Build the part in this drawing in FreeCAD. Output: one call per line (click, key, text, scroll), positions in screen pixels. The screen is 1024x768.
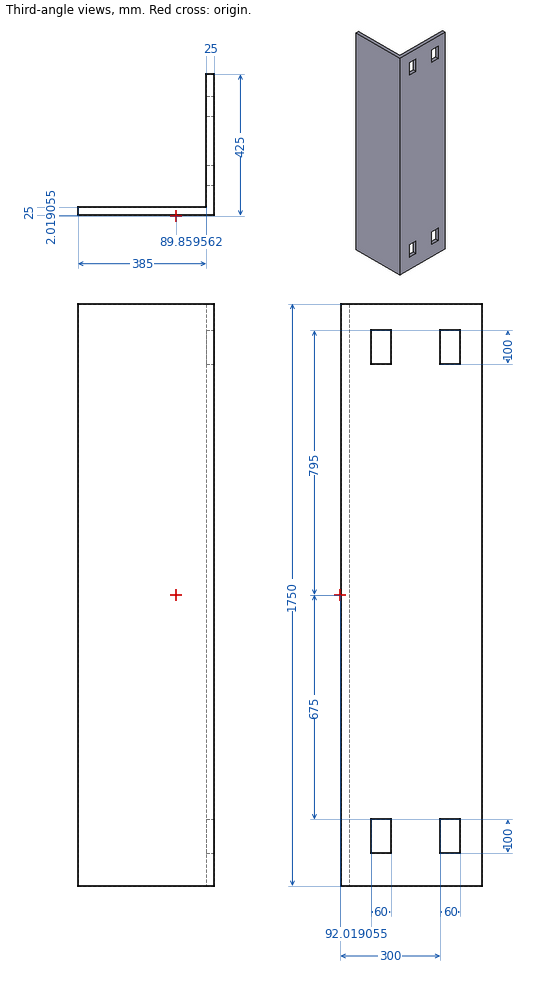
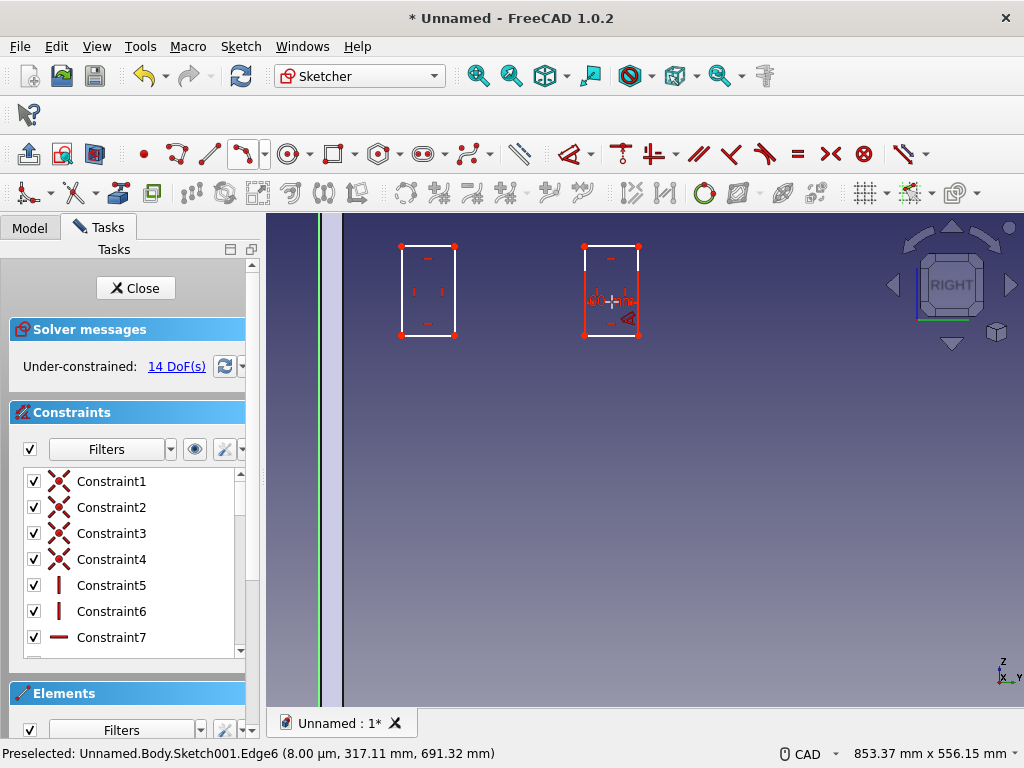
scroll(601, 338, down, 8)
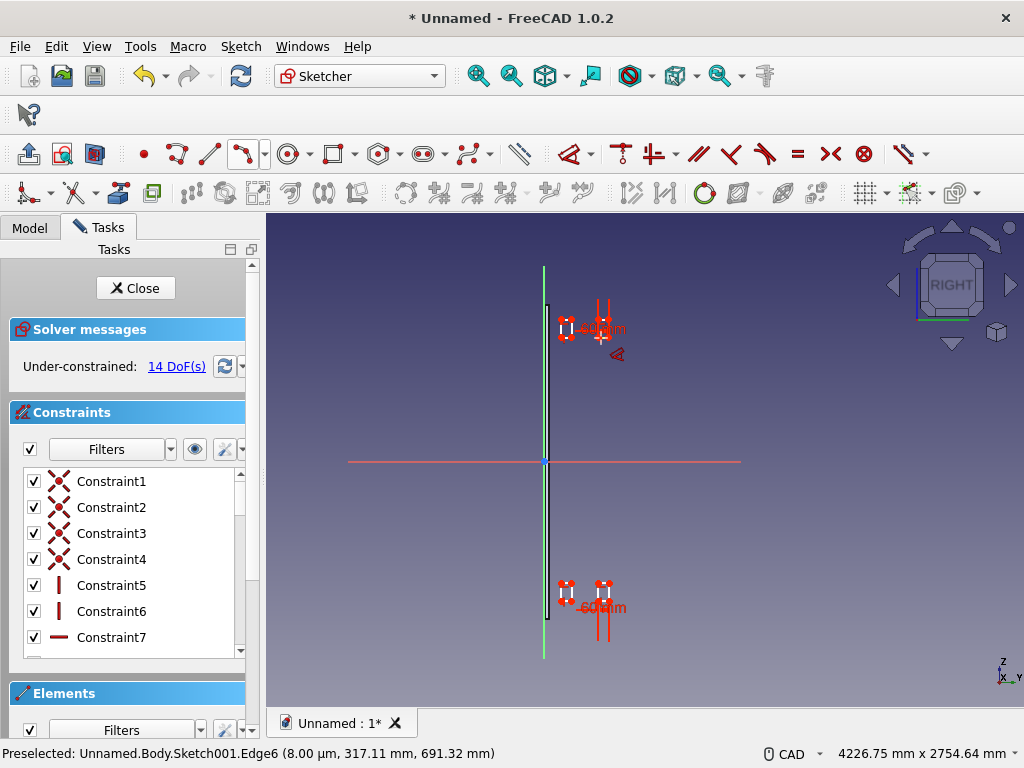
scroll(564, 601, up, 8)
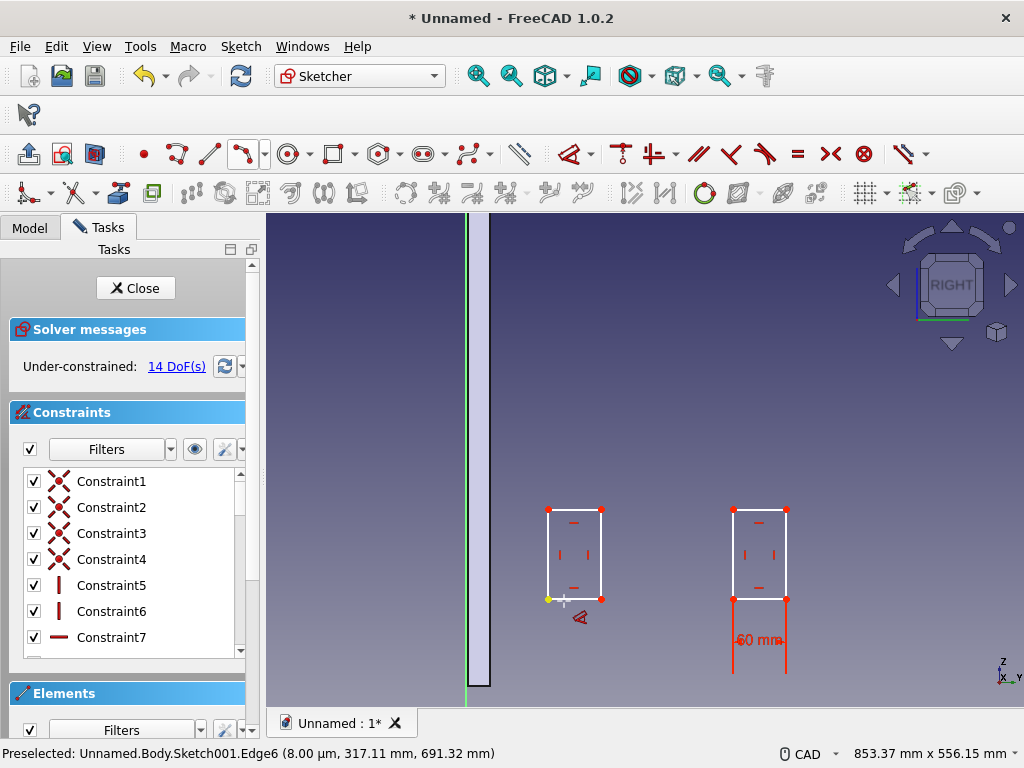
click(564, 599)
click(575, 633)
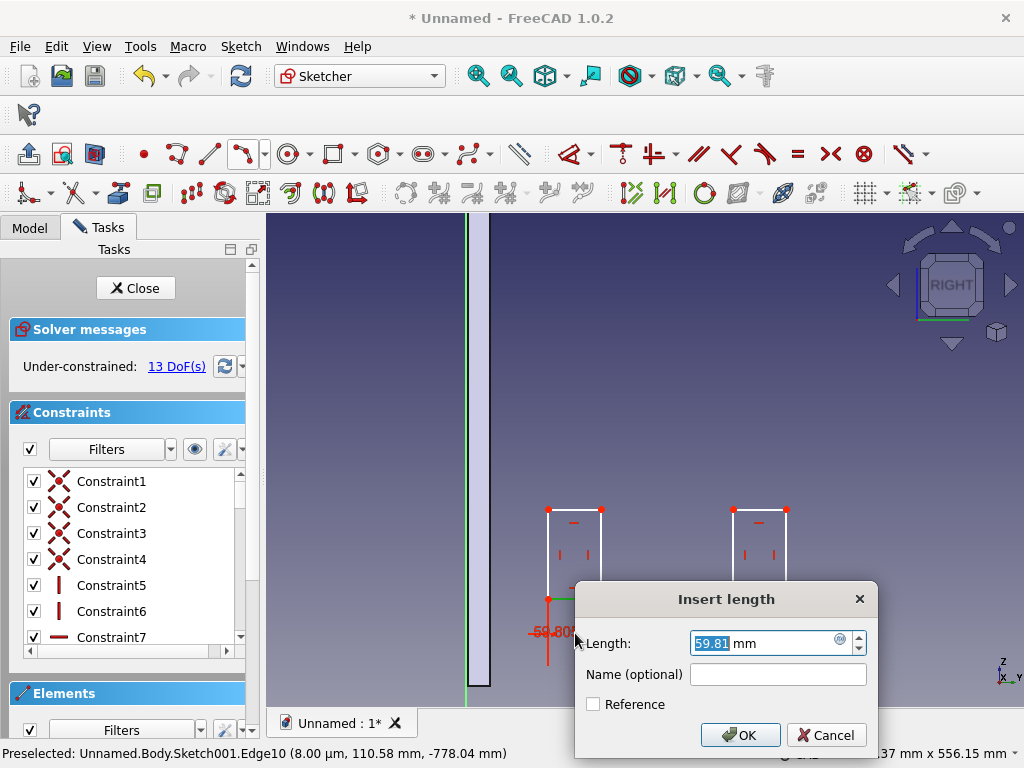
text(60)
key(Return)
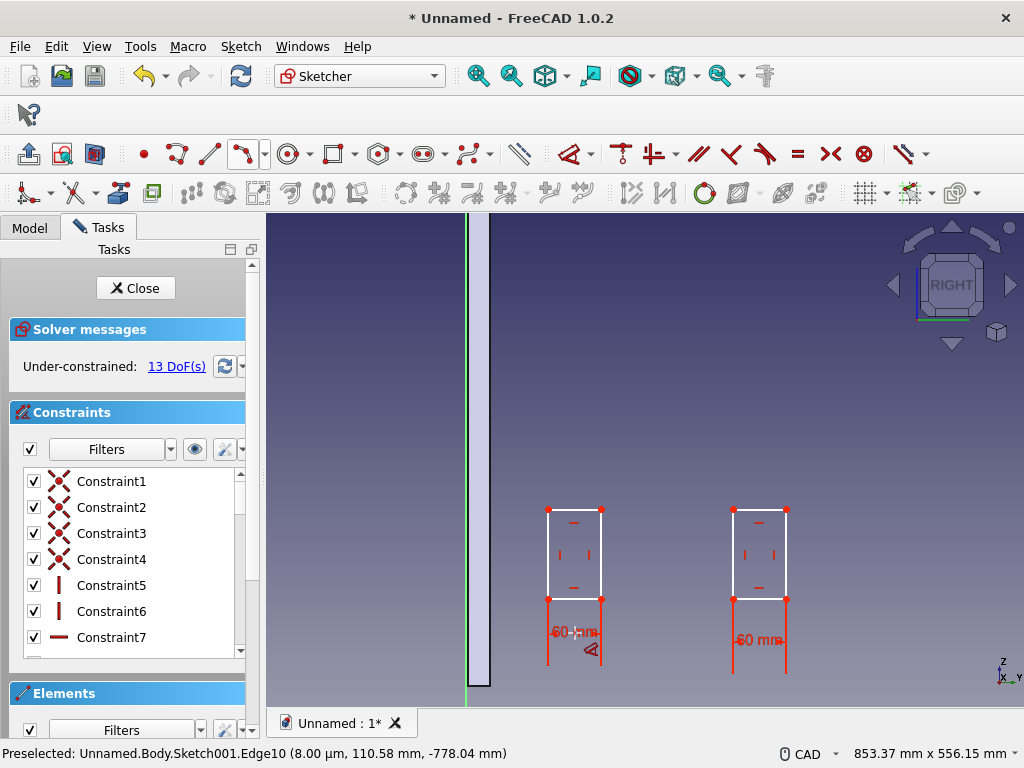
scroll(564, 602, down, 8)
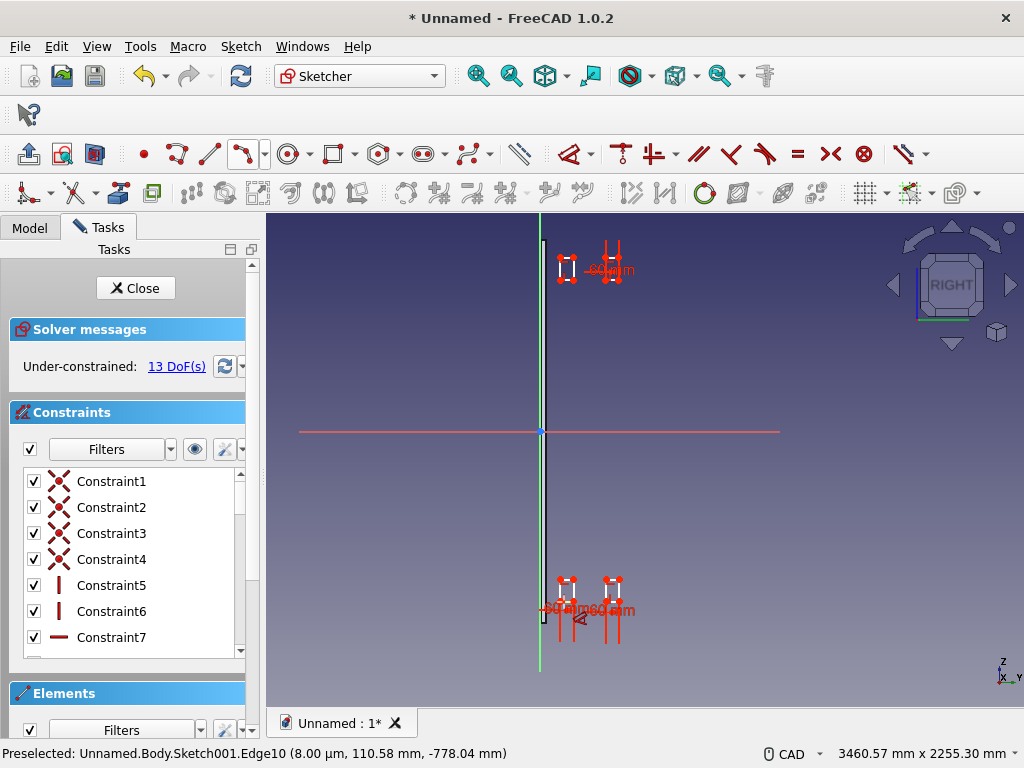
scroll(564, 339, up, 8)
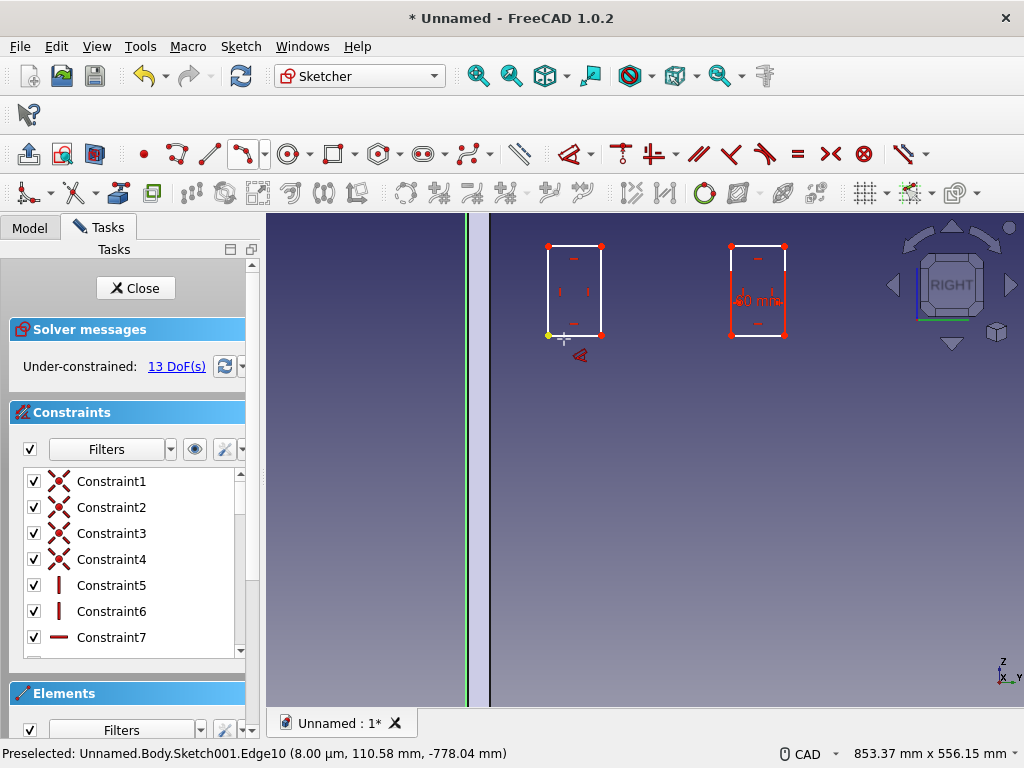
click(564, 336)
click(575, 302)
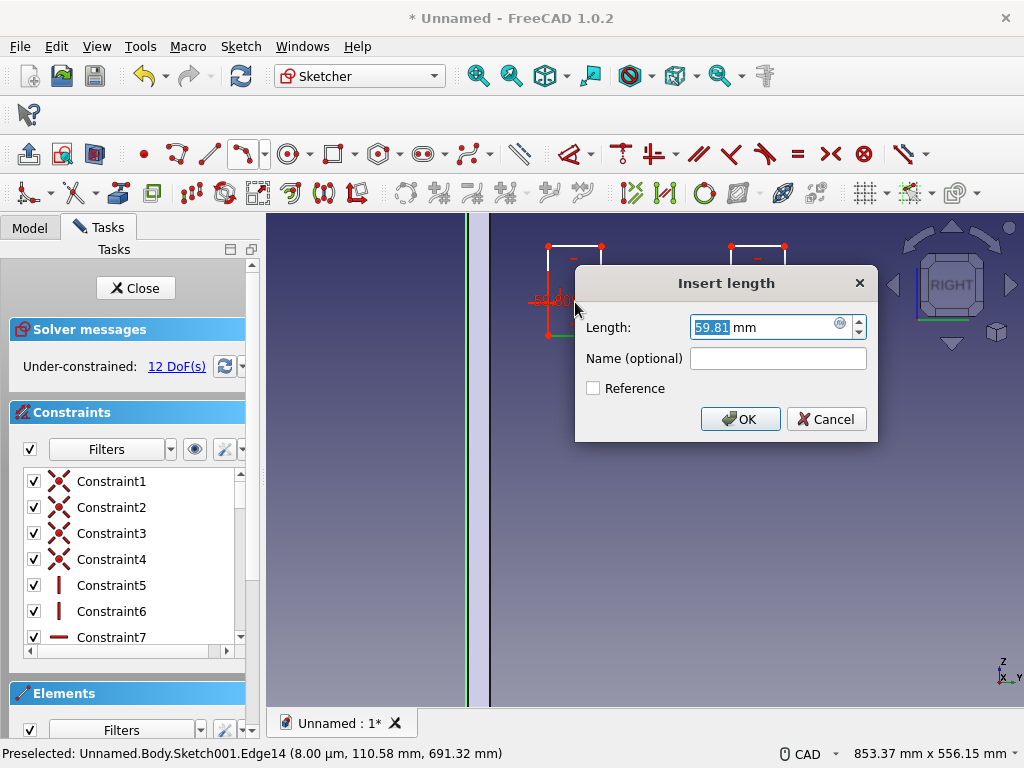
text(60)
key(Return)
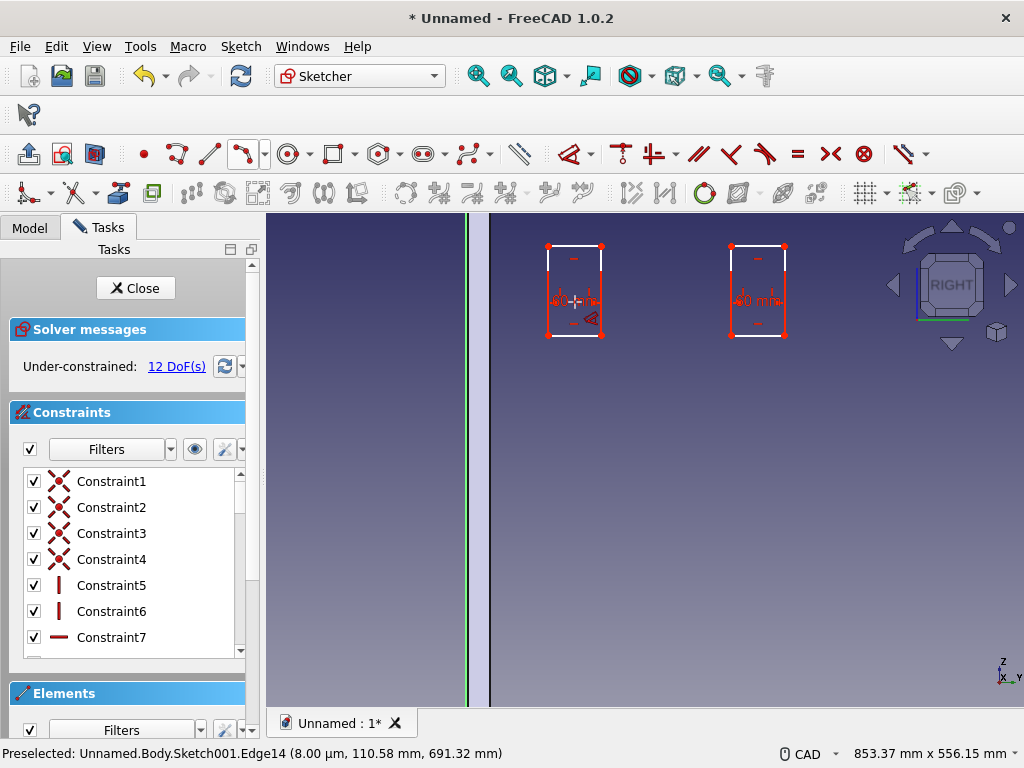
scroll(564, 338, down, 8)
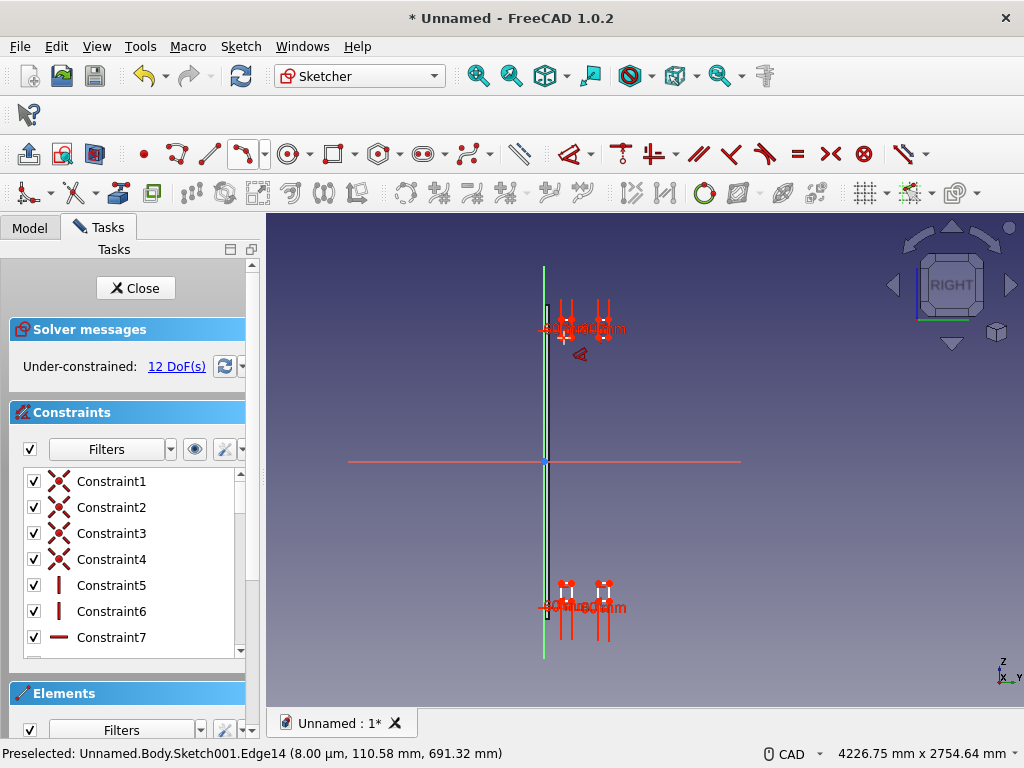
scroll(598, 589, up, 5)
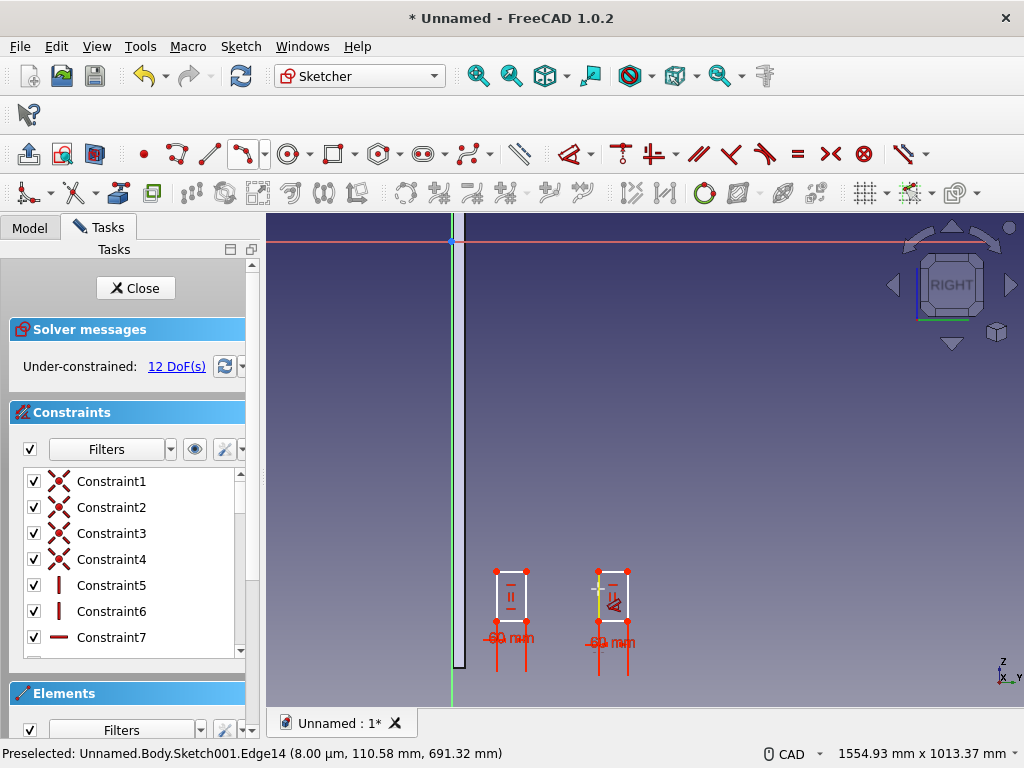
click(599, 587)
click(565, 597)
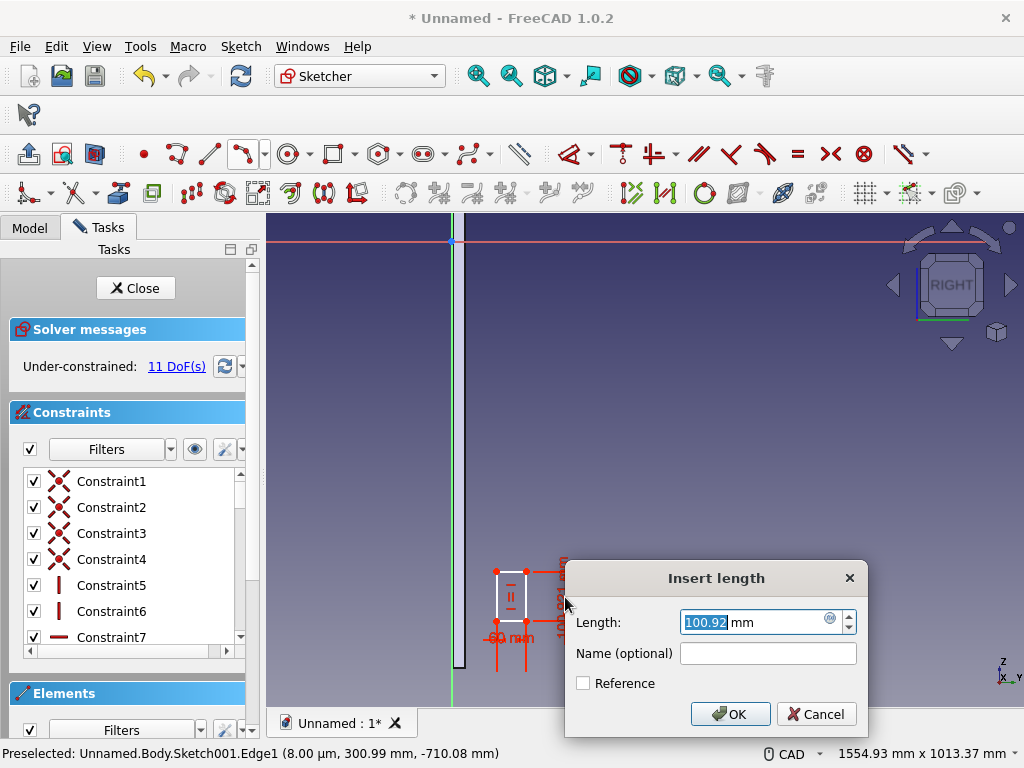
text(100)
key(Return)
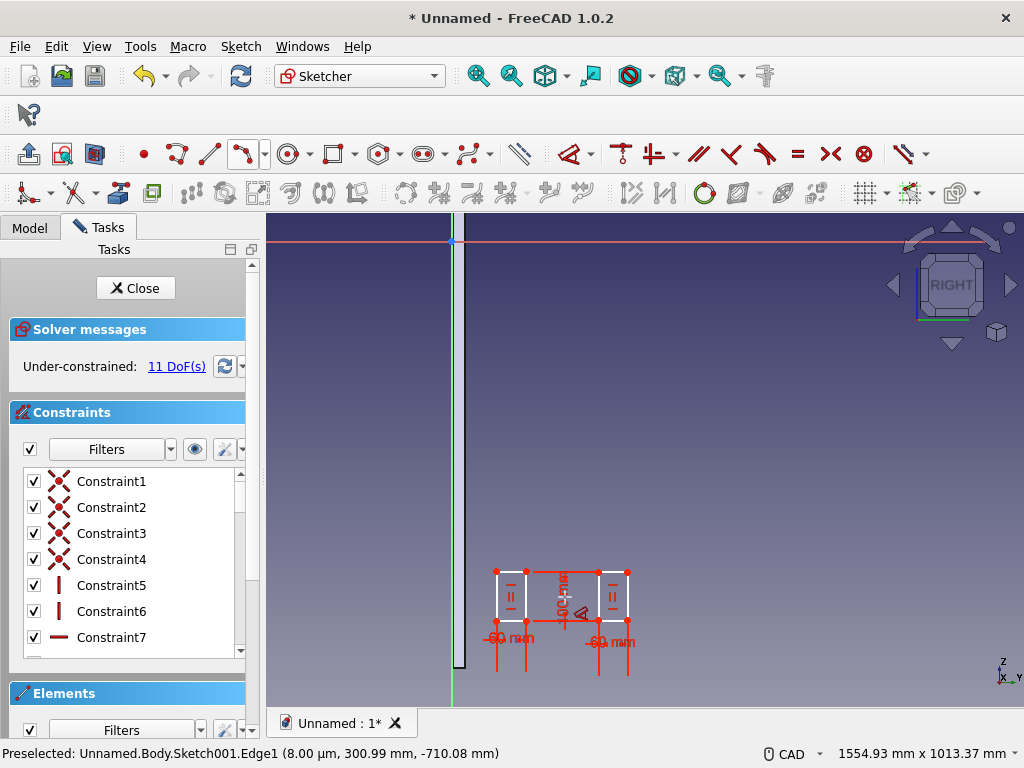
scroll(598, 590, down, 5)